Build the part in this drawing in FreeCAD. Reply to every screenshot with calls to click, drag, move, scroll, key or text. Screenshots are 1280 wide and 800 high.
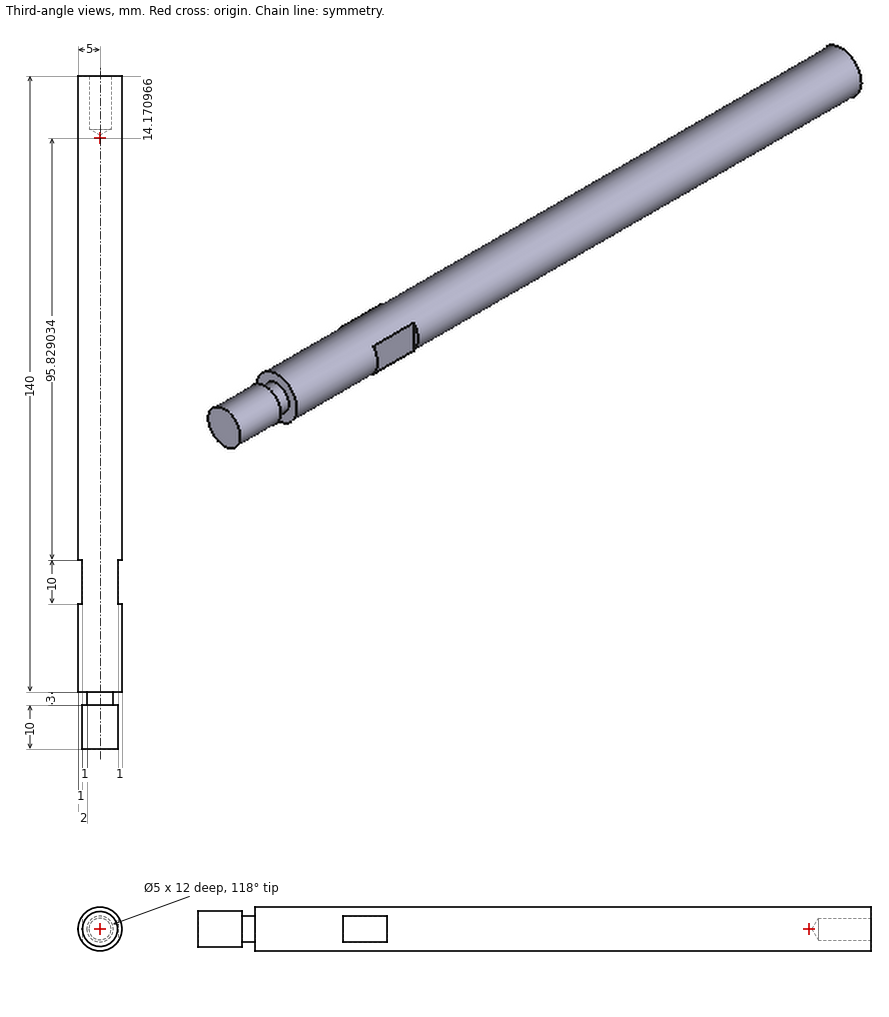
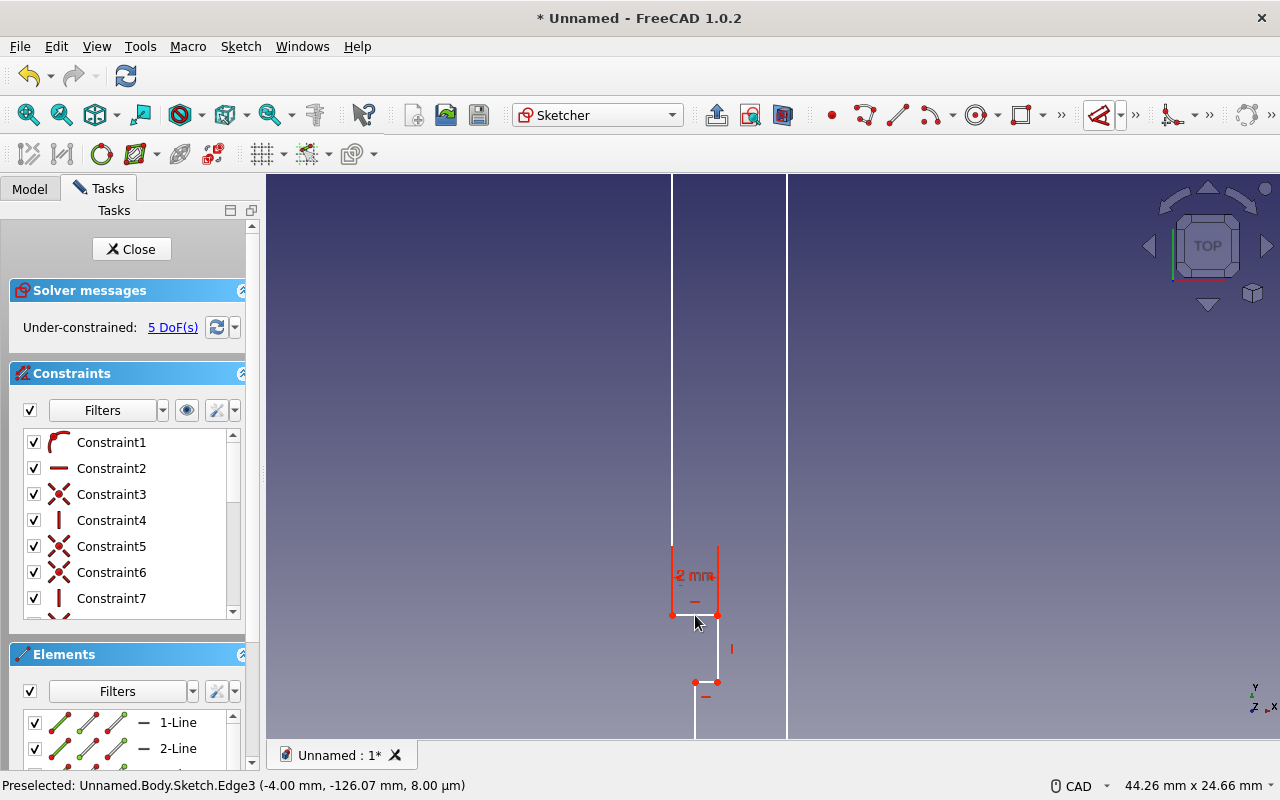
click(718, 635)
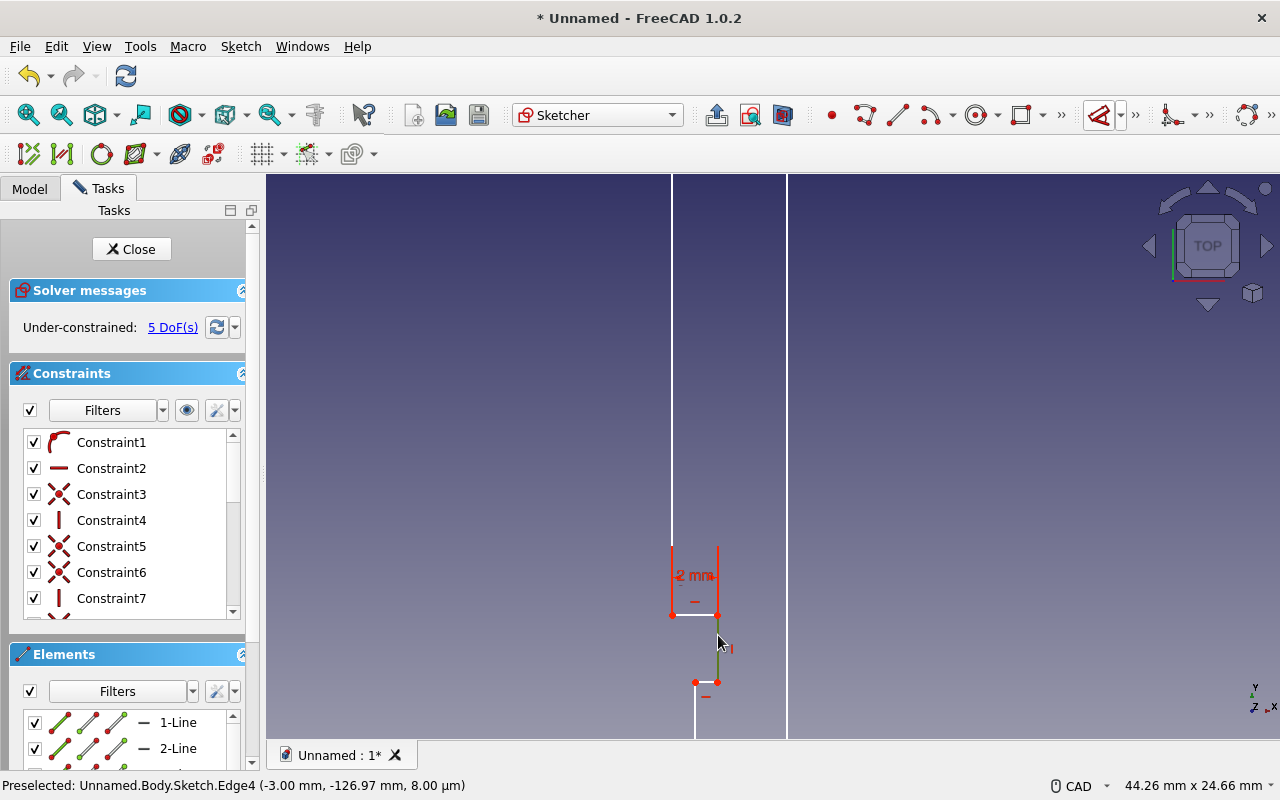
click(1120, 116)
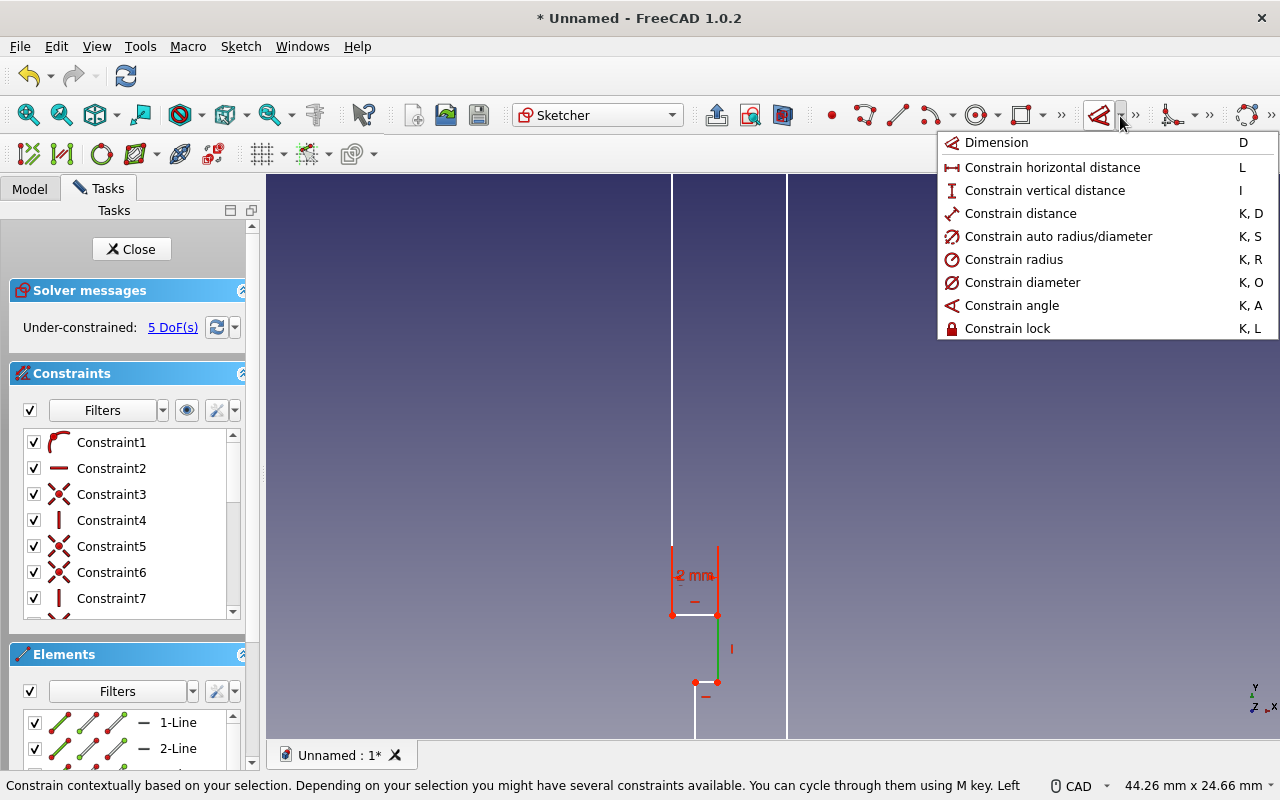
click(1108, 190)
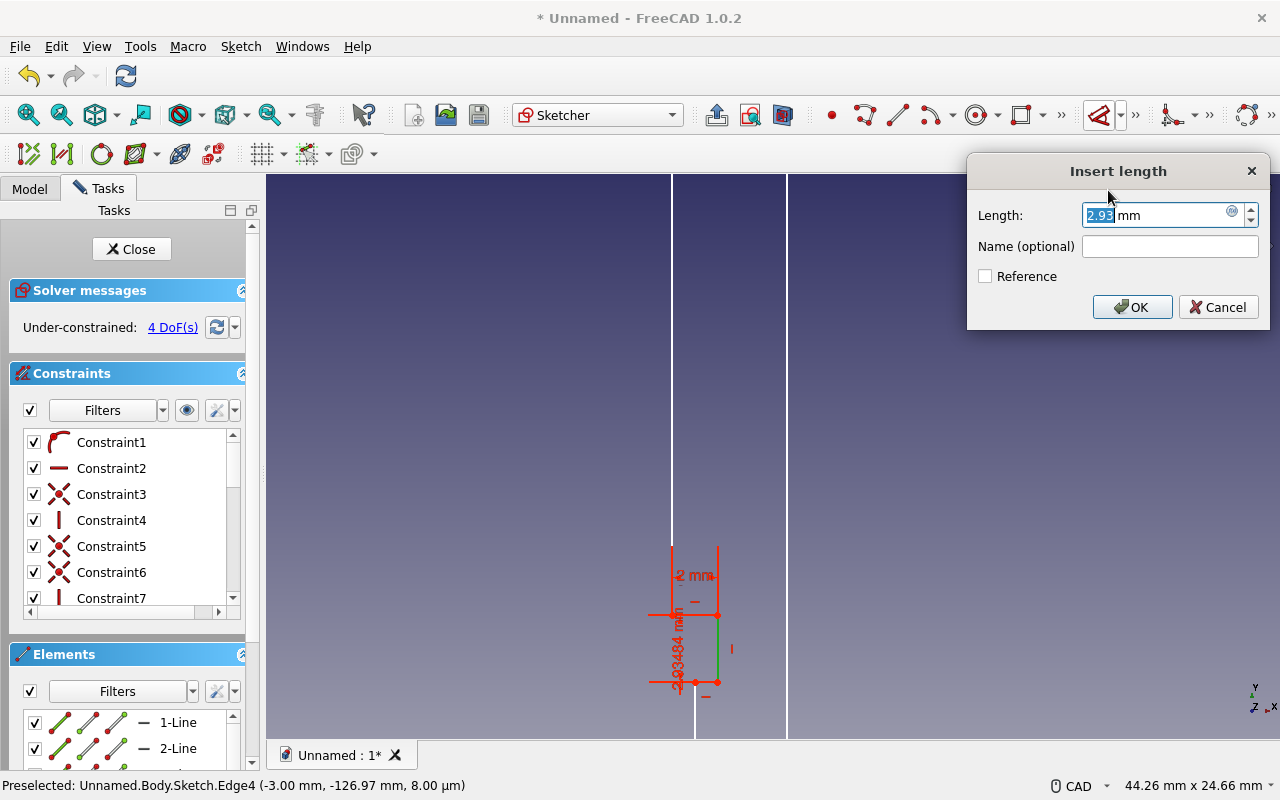
text(3)
key(Return)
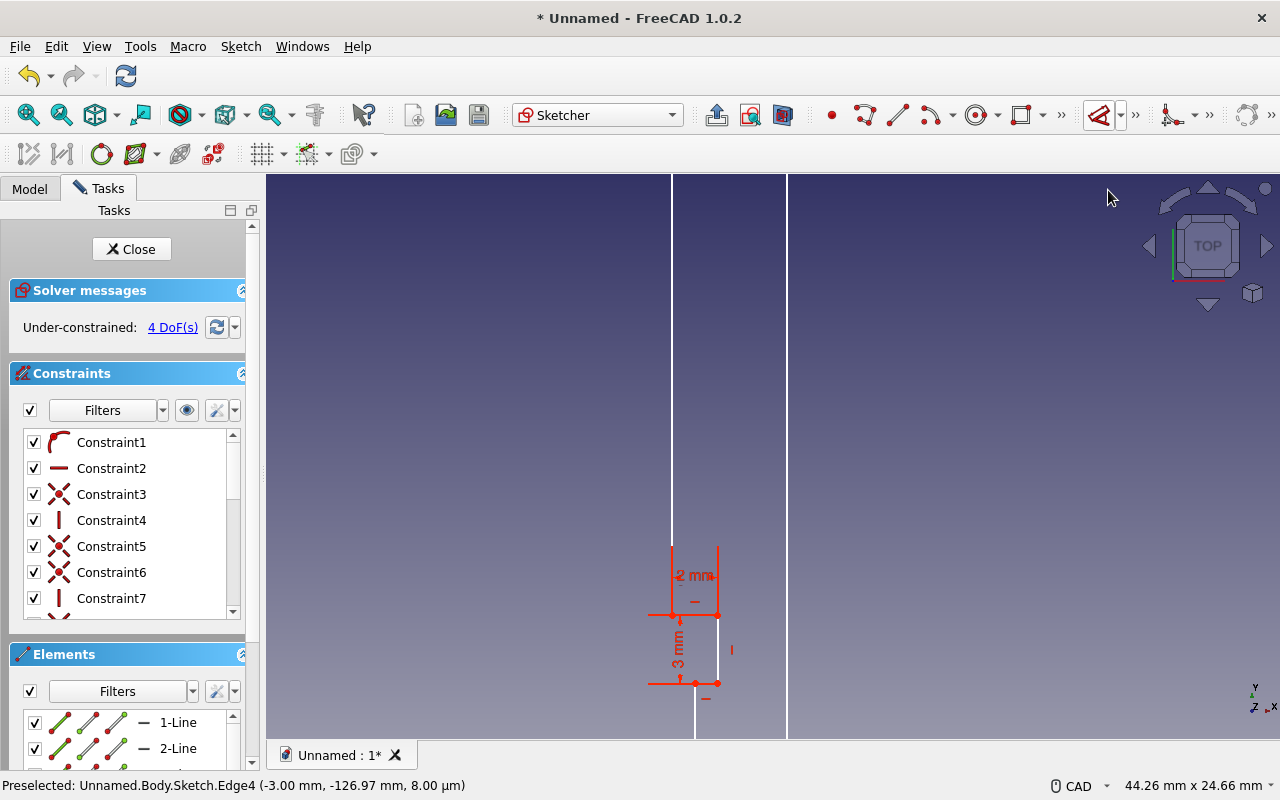
scroll(707, 684, up, 3)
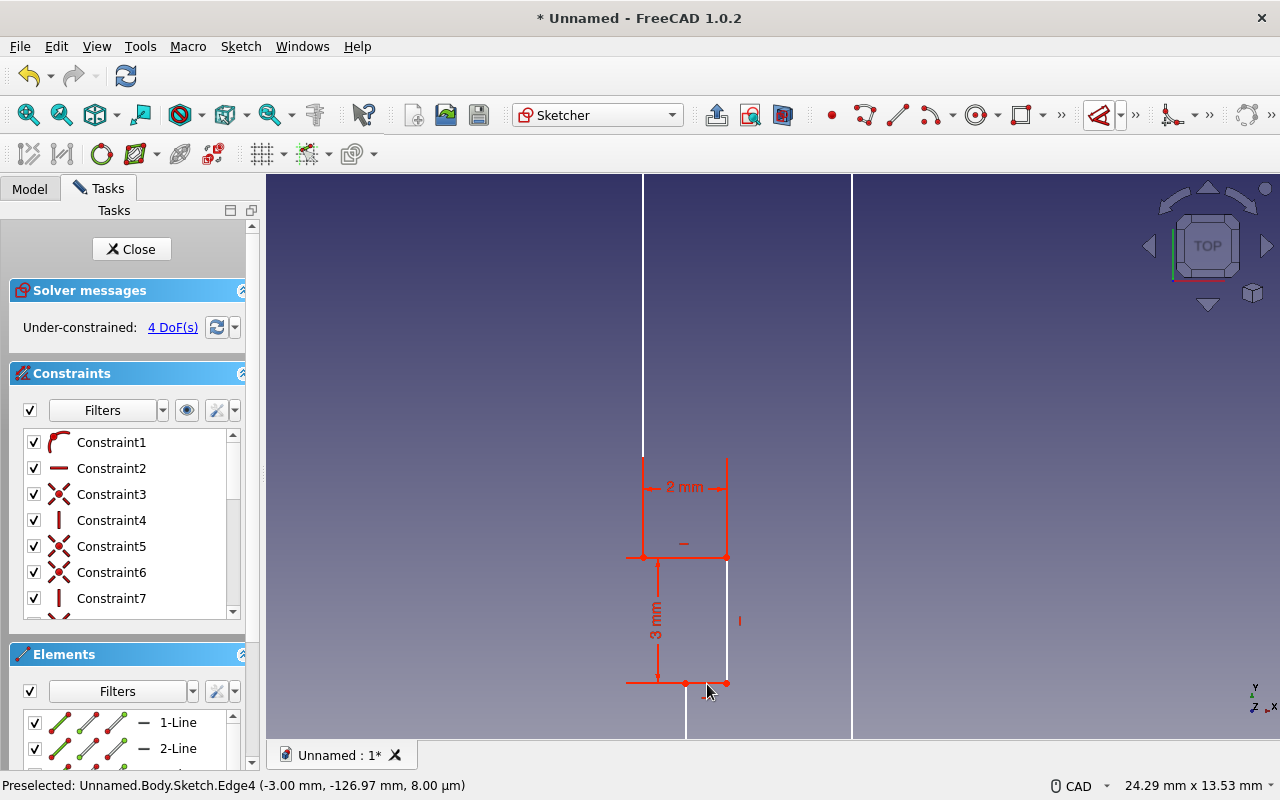
click(706, 683)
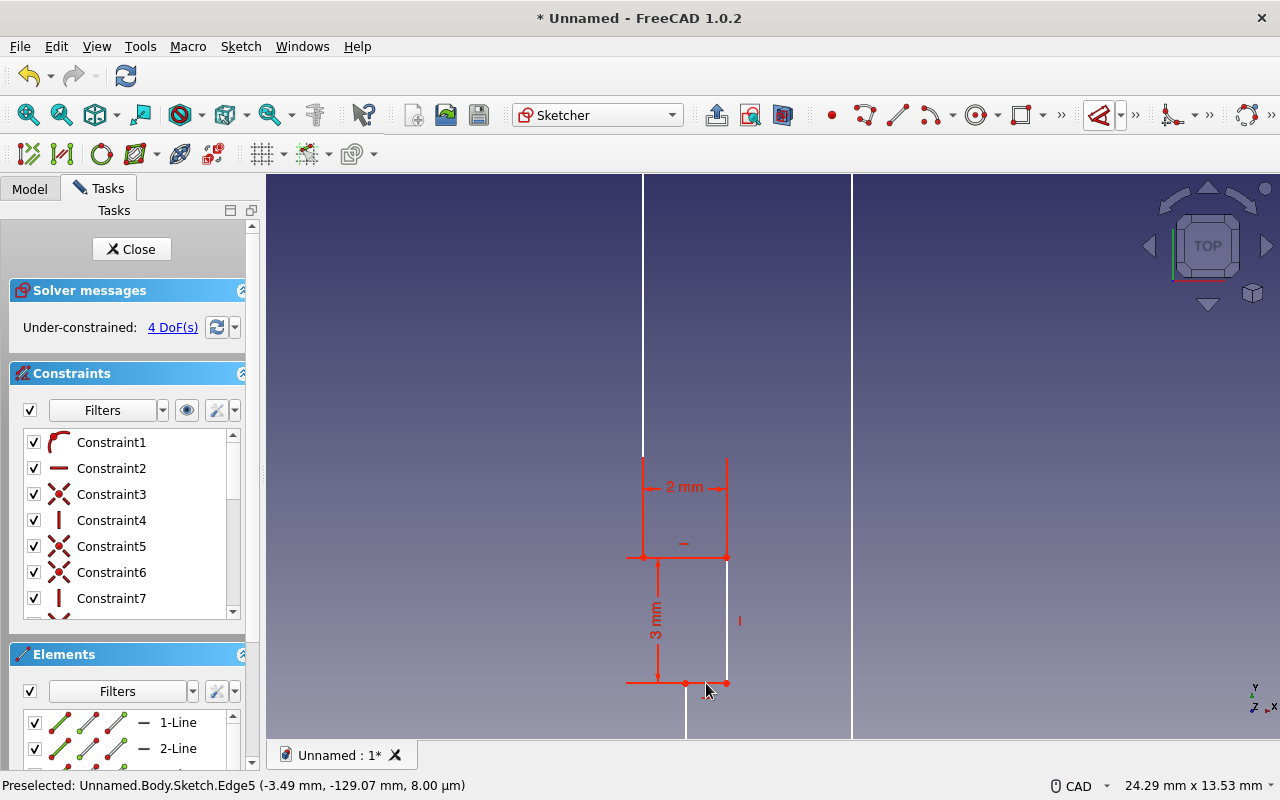
key(l)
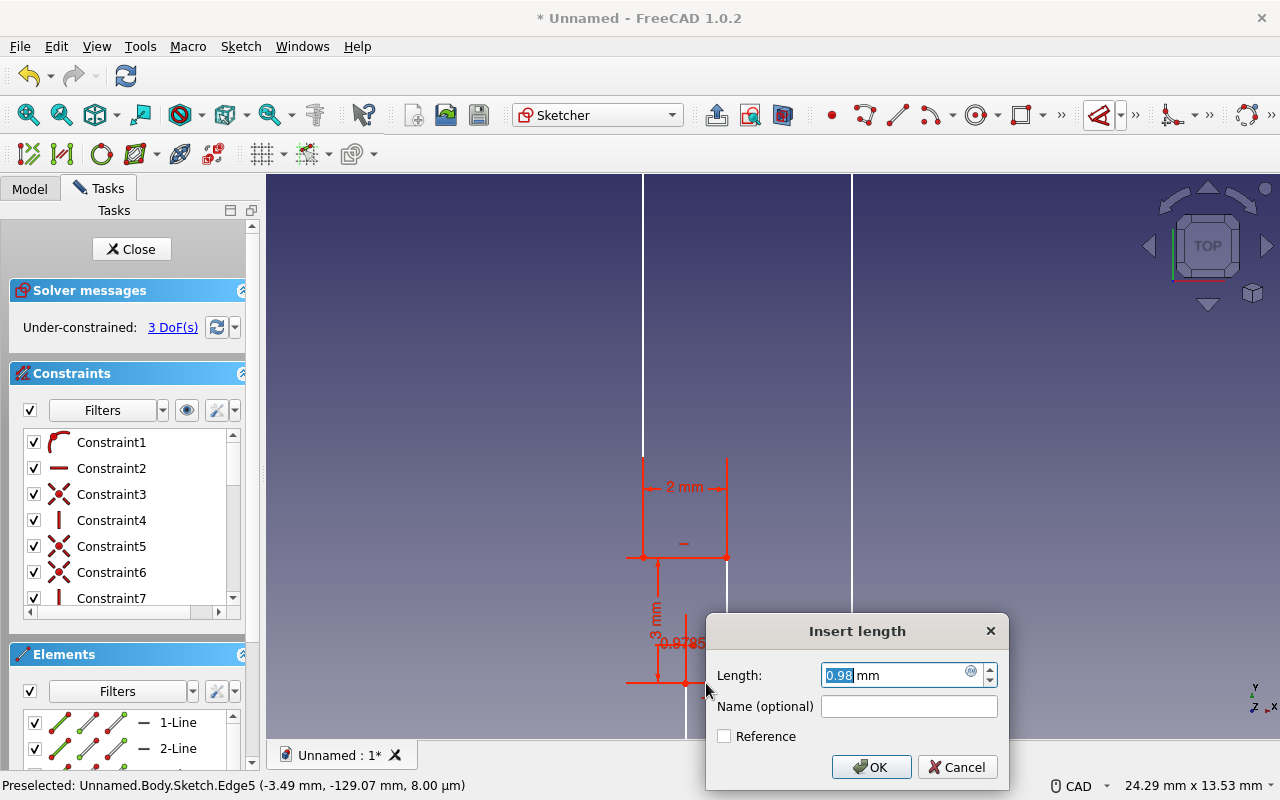
text(1)
key(Return)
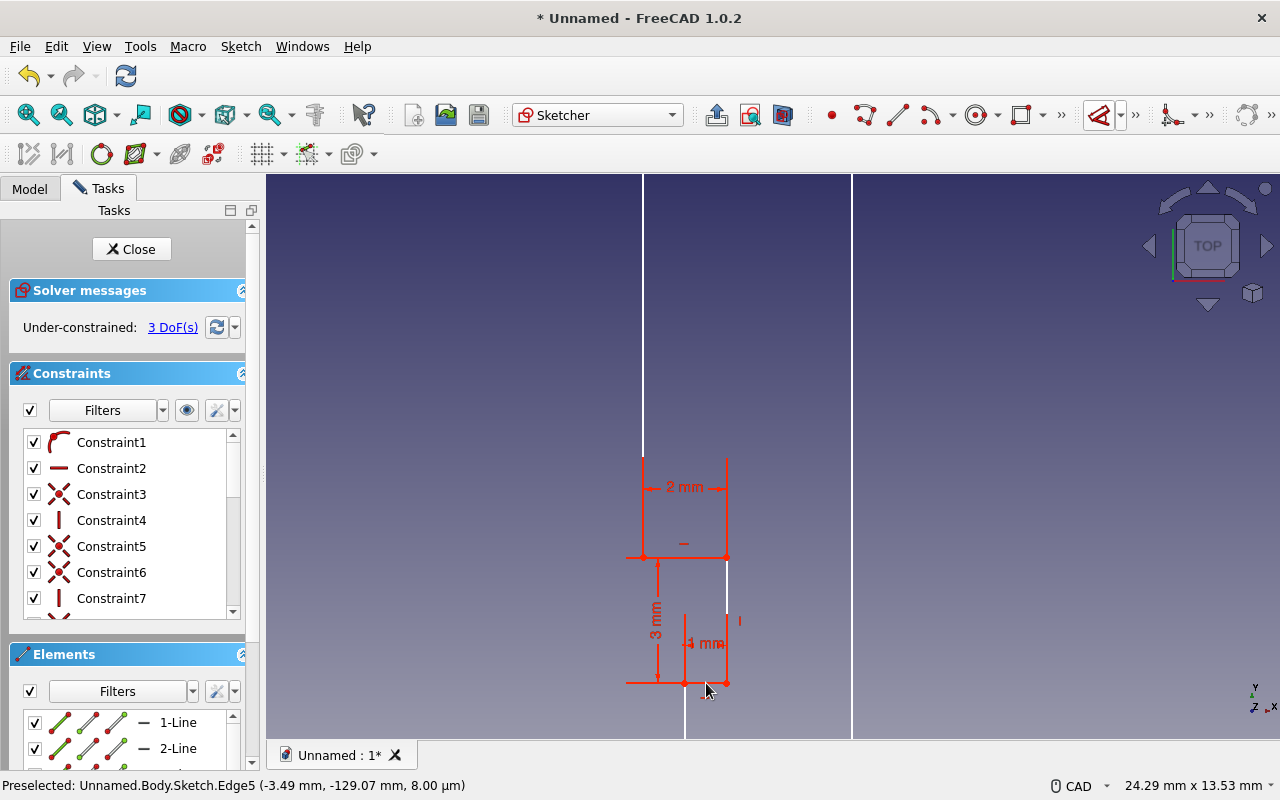
scroll(702, 622, down, 14)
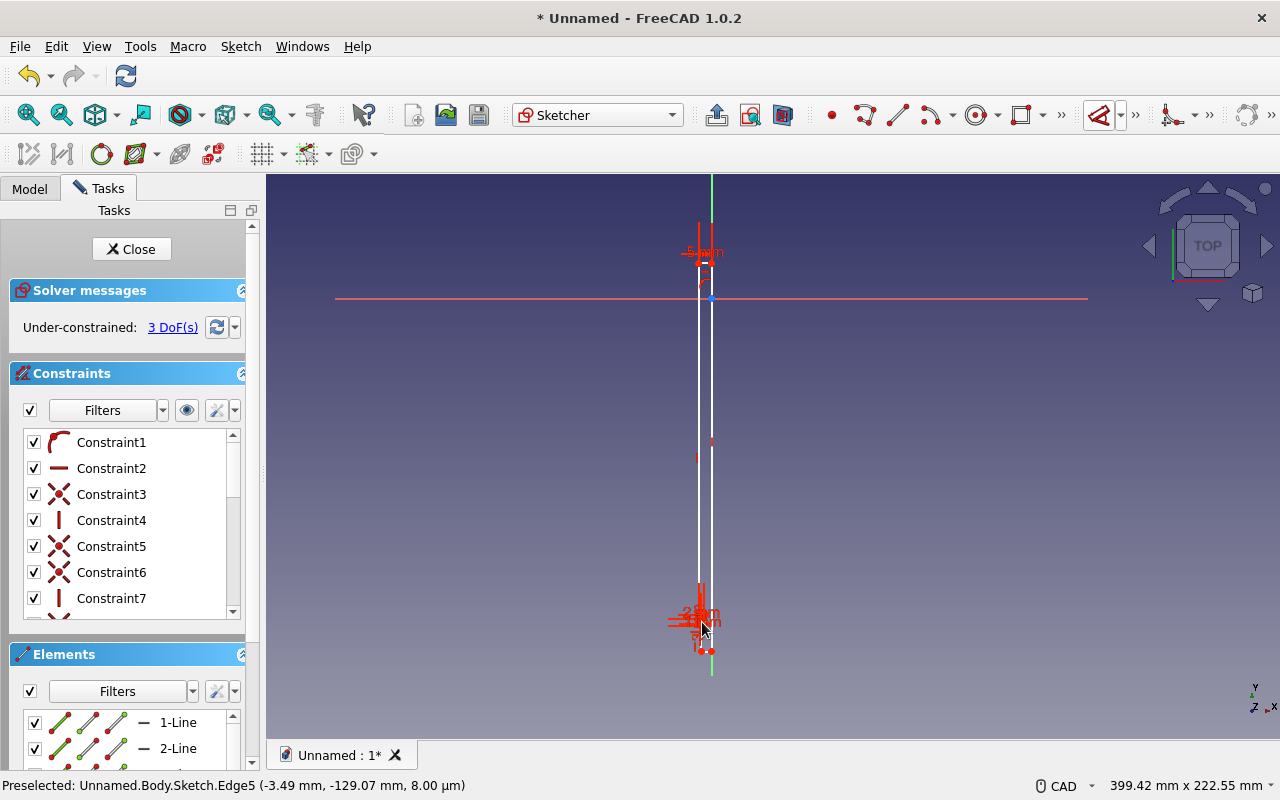
scroll(701, 634, up, 3)